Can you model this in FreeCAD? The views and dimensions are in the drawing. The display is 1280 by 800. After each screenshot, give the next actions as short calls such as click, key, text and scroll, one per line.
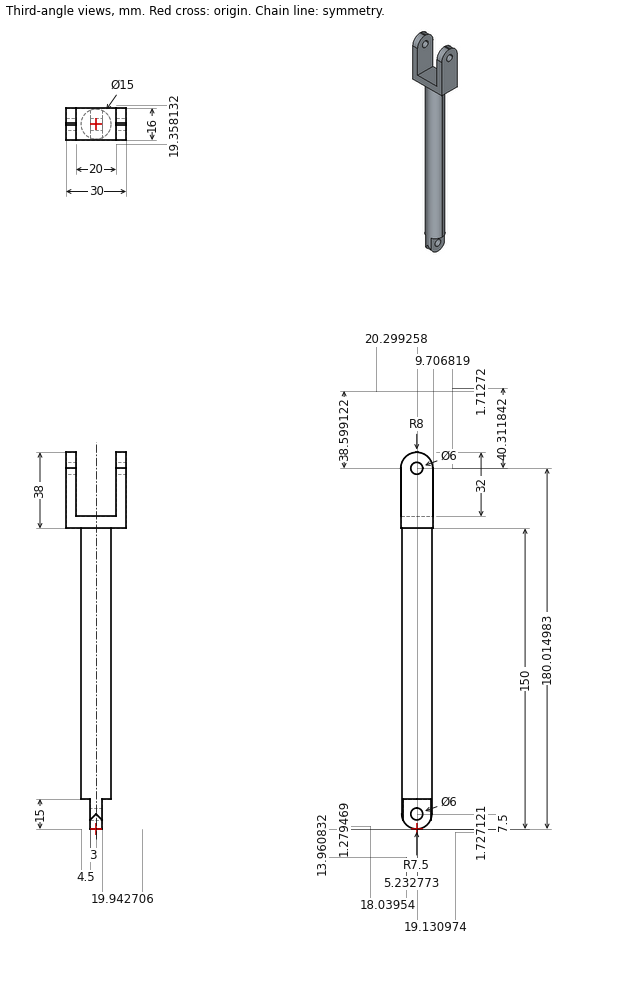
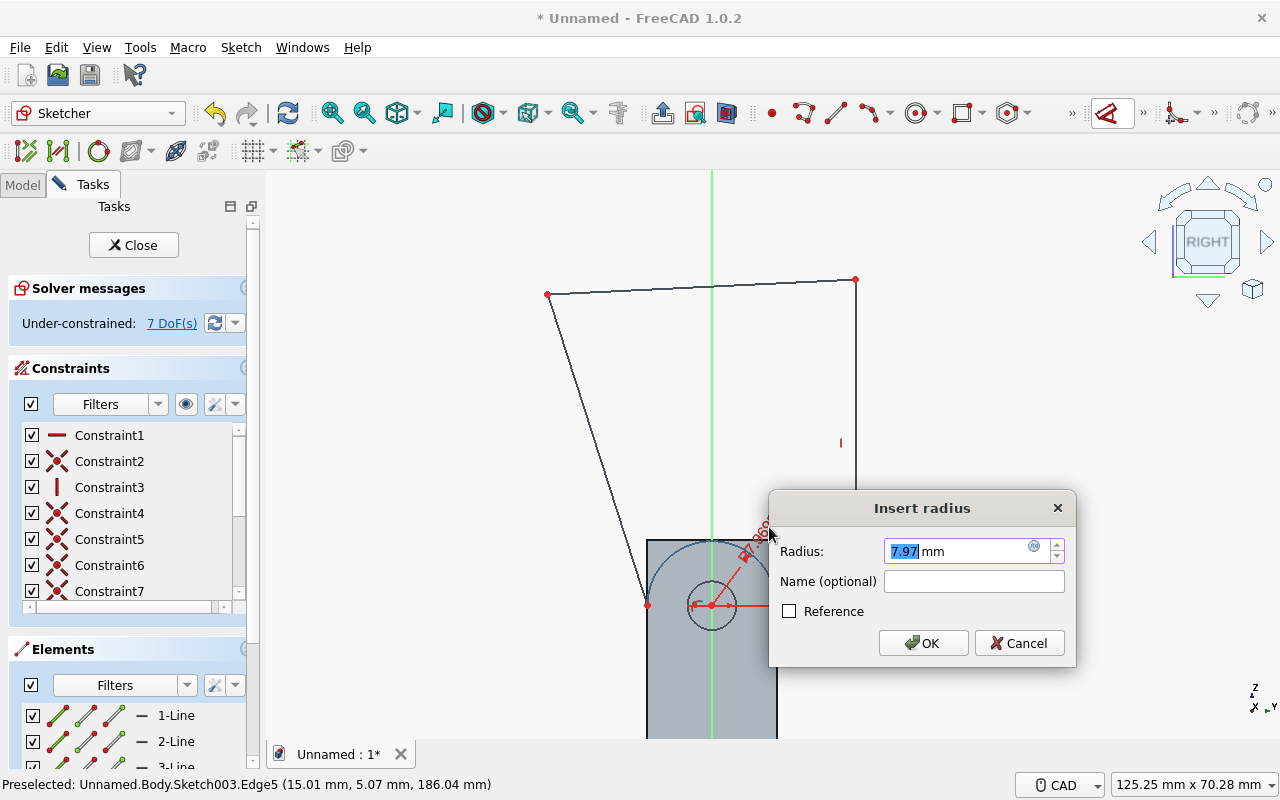
text(8)
key(Return)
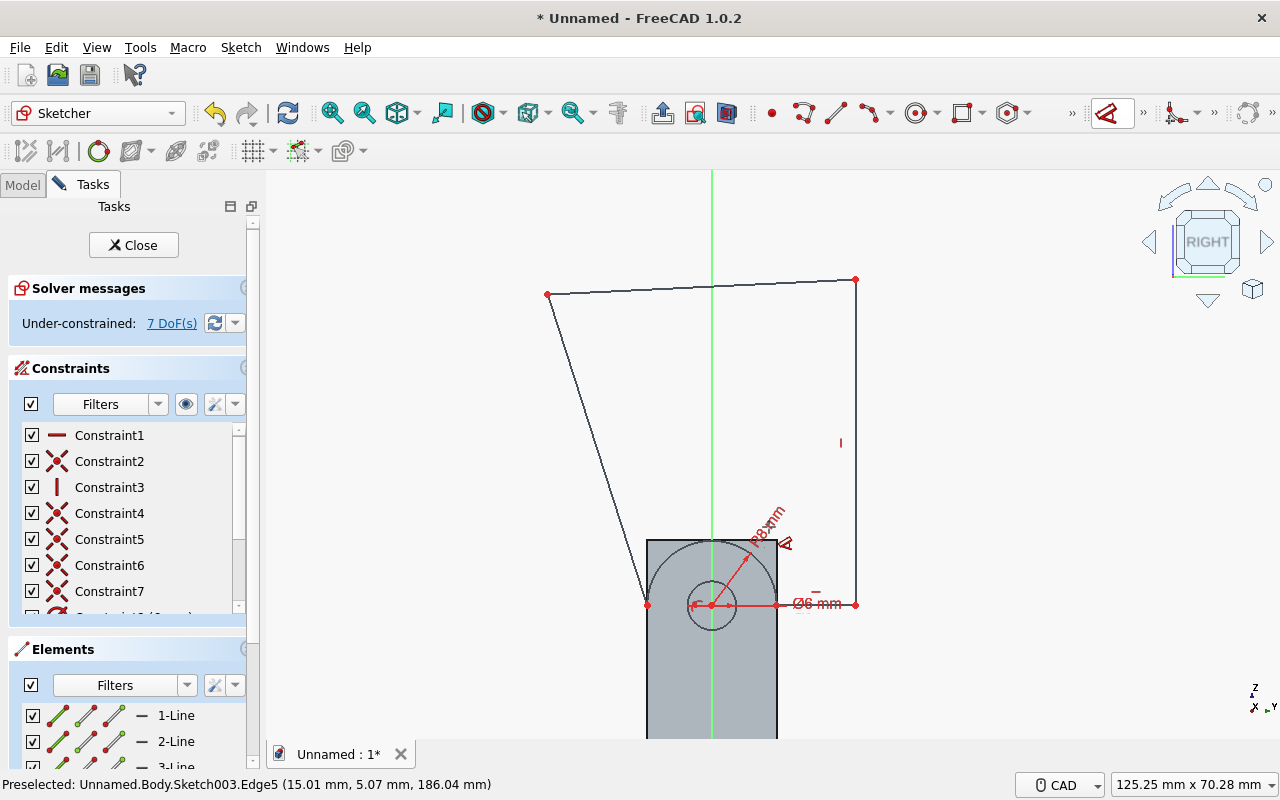
click(800, 605)
click(816, 639)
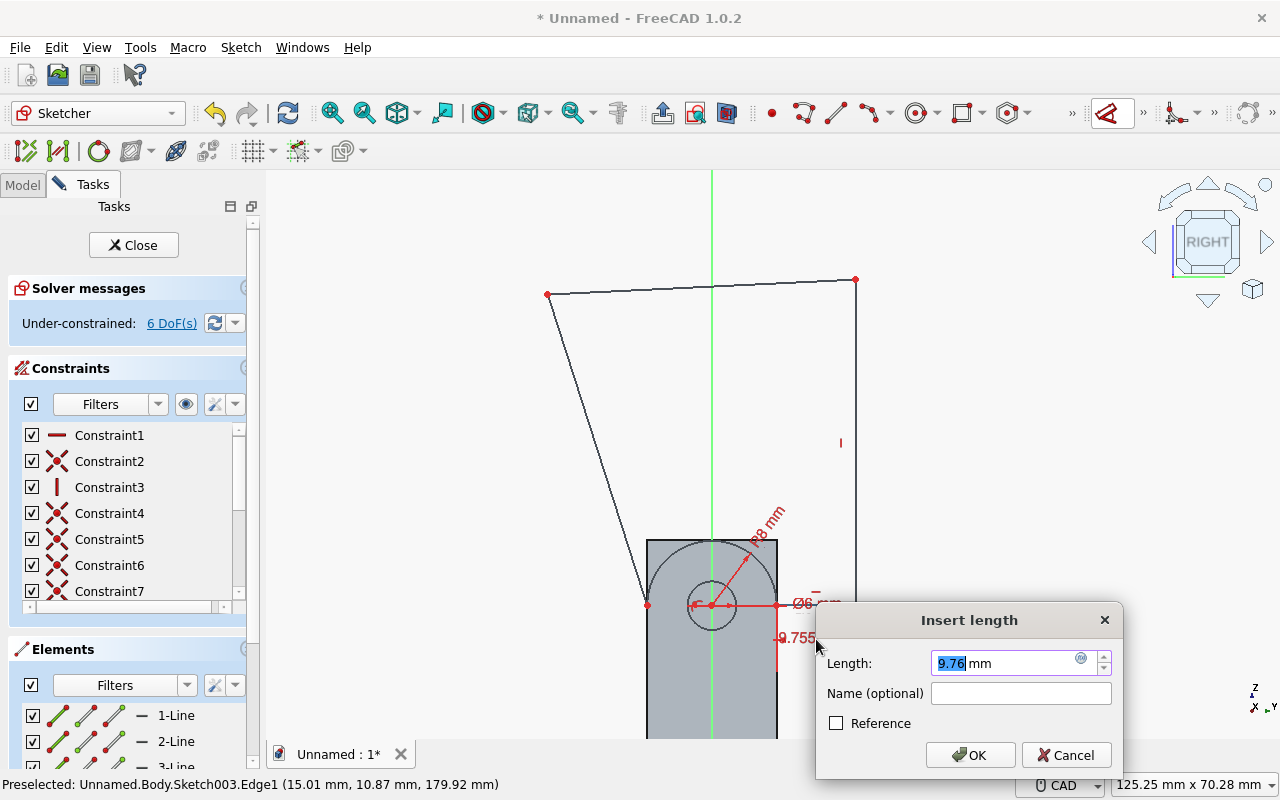
text(9.706819)
key(Return)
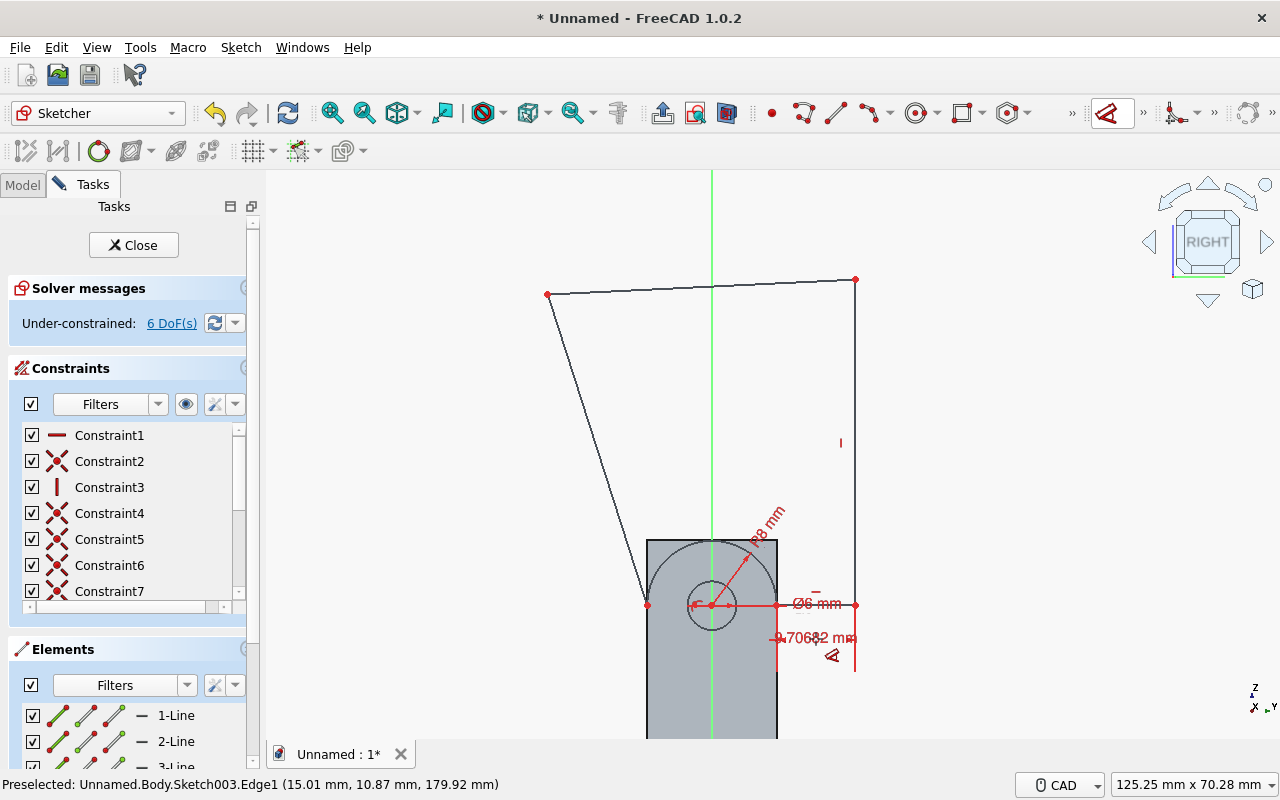
scroll(763, 284, up, 6)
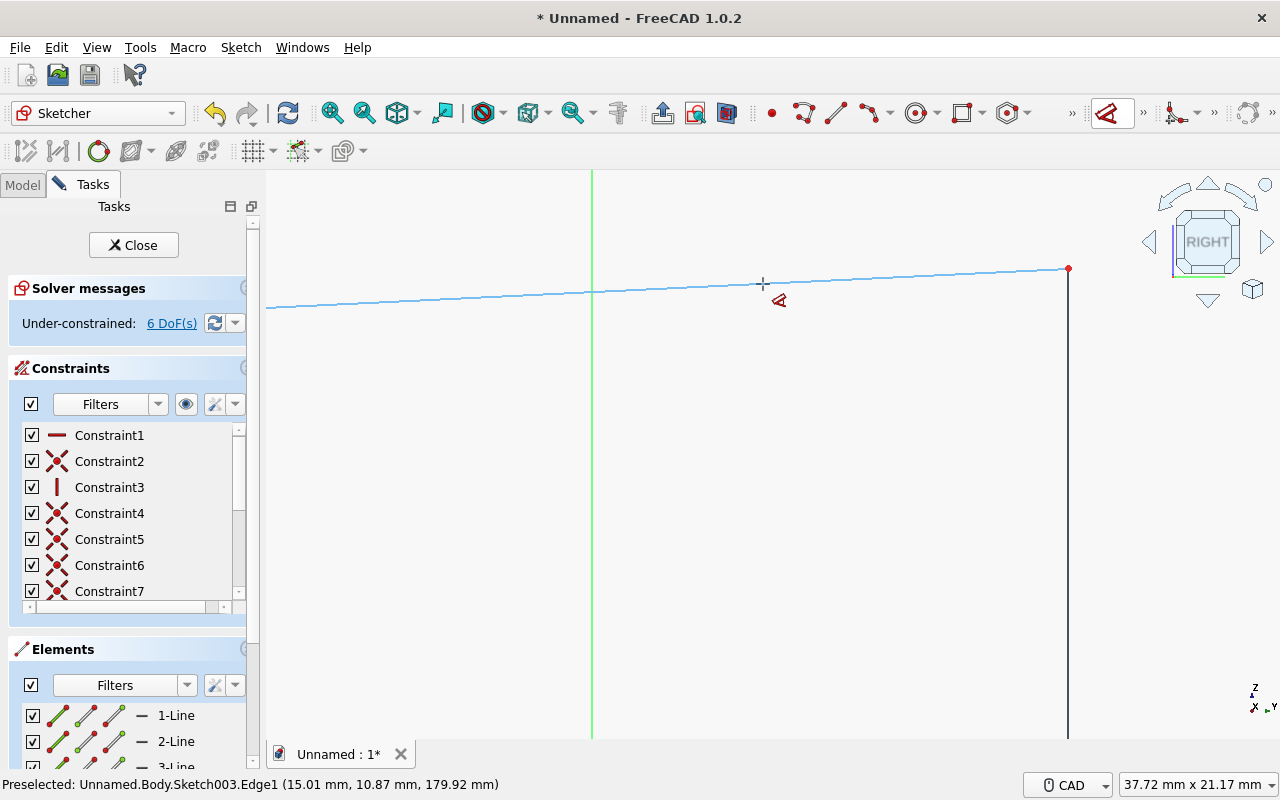
click(762, 284)
click(1102, 294)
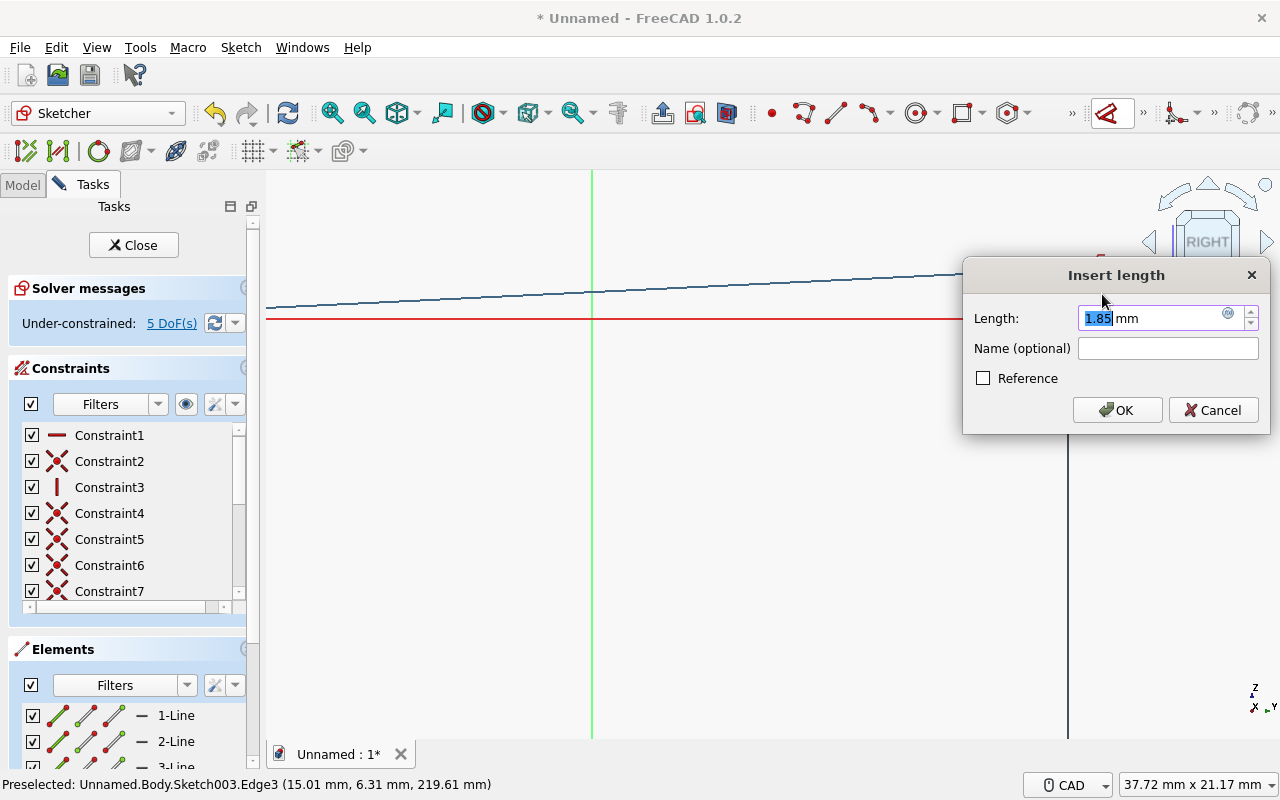
text(1.71272)
key(Return)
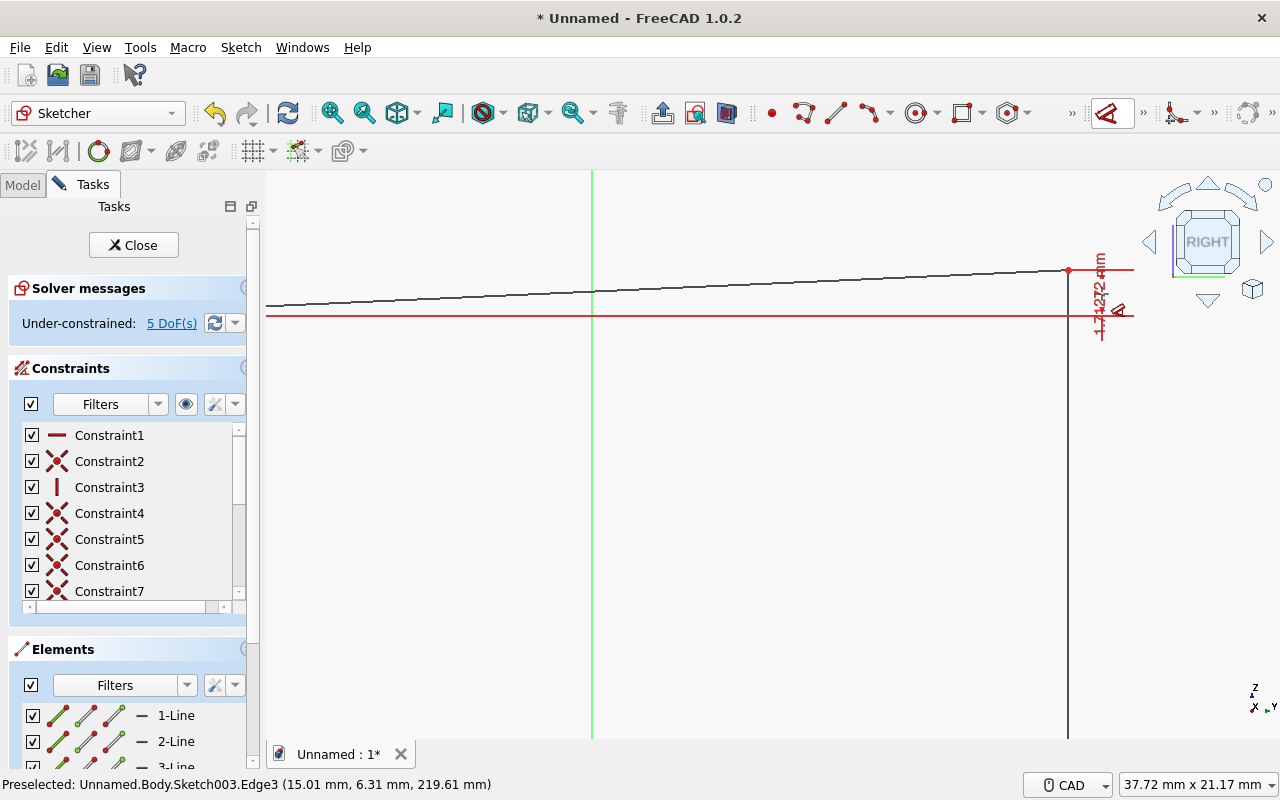
click(1068, 594)
click(1102, 491)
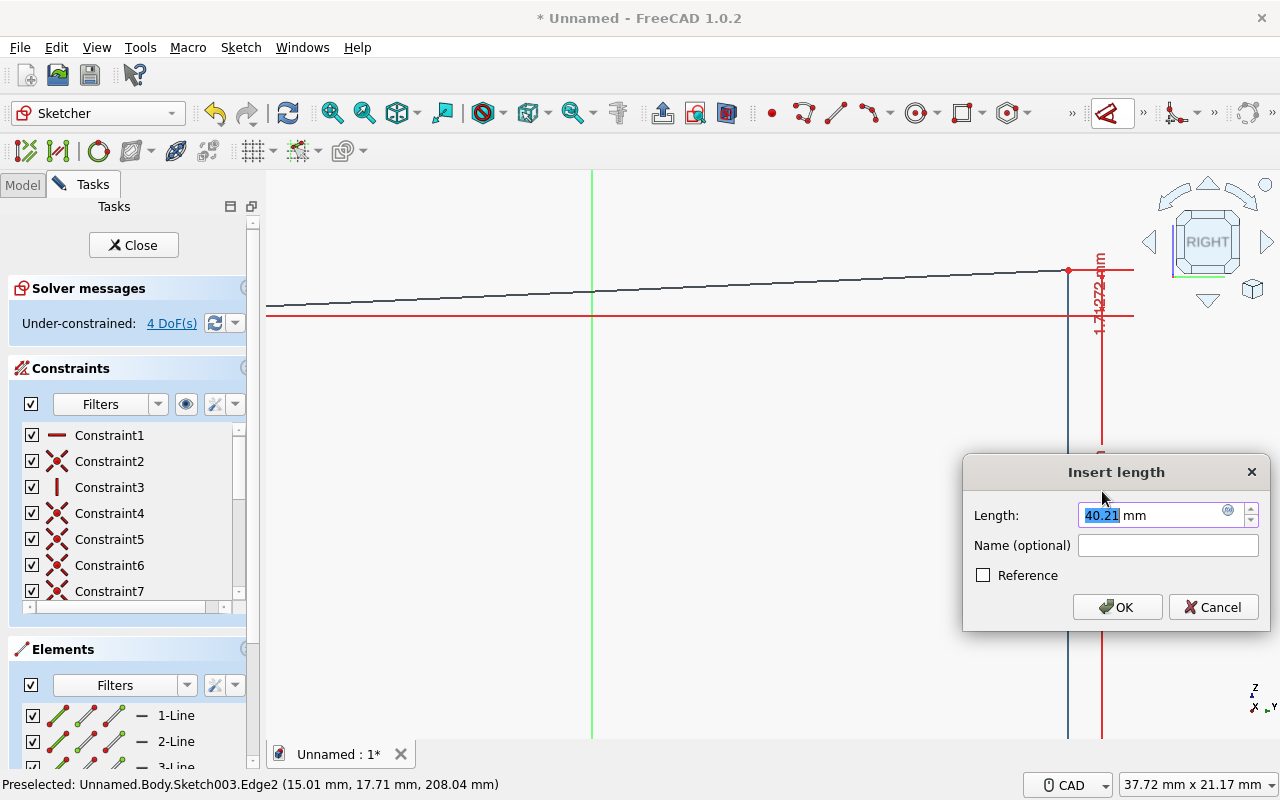
text(40.311842)
key(Return)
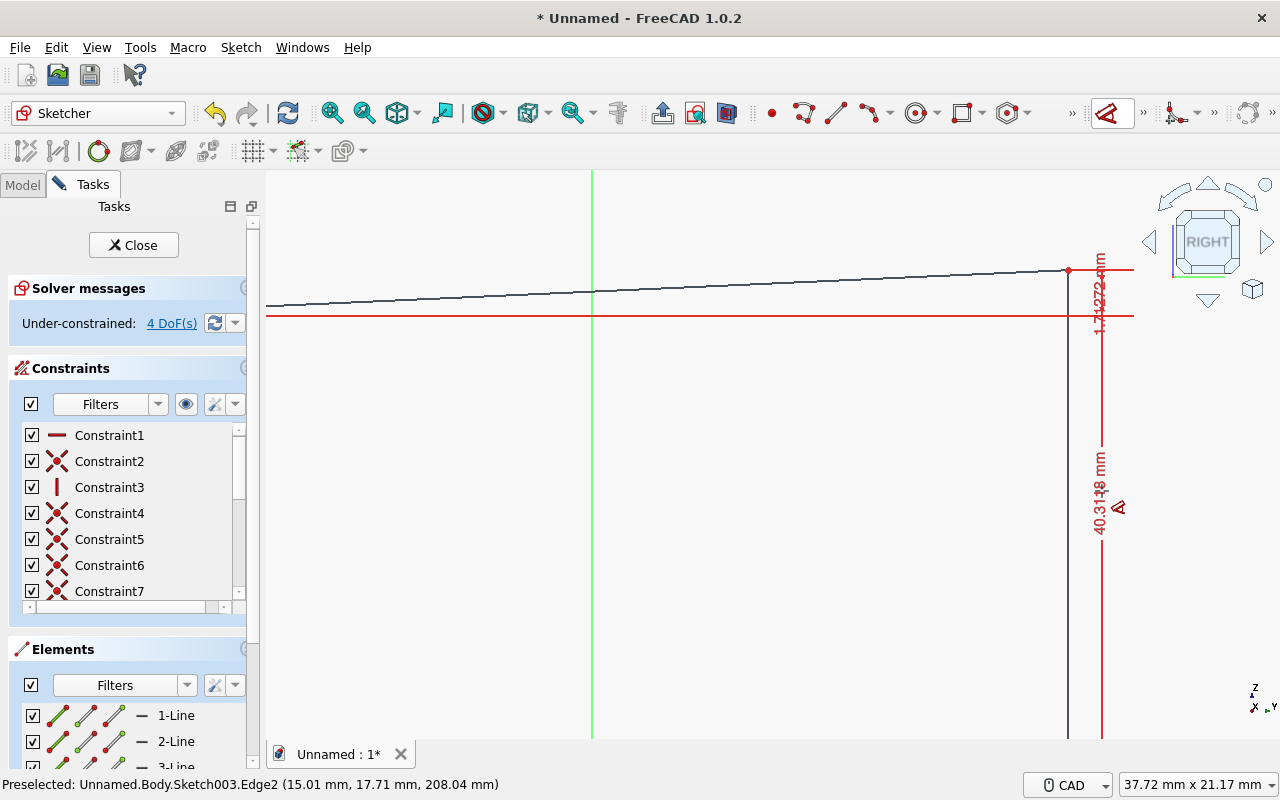
scroll(768, 285, down, 6)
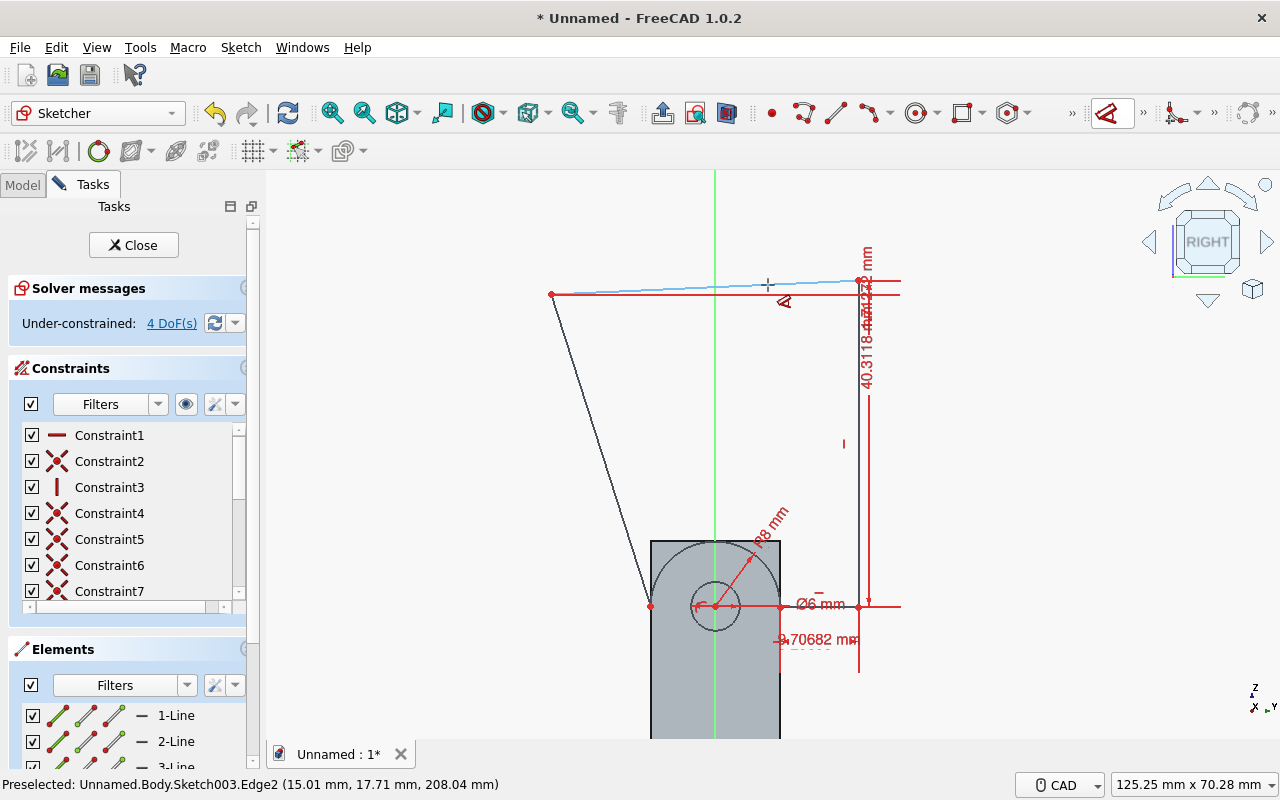
click(551, 295)
click(633, 261)